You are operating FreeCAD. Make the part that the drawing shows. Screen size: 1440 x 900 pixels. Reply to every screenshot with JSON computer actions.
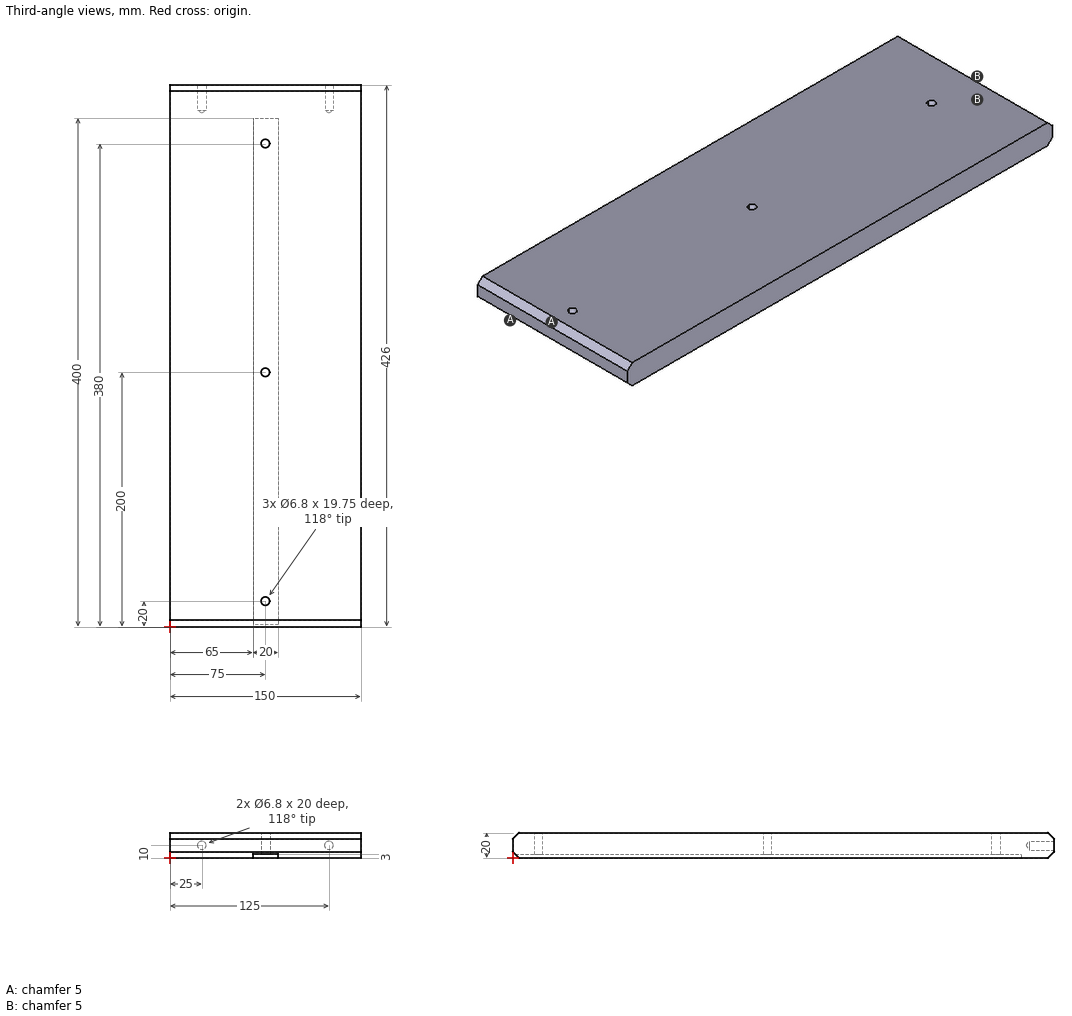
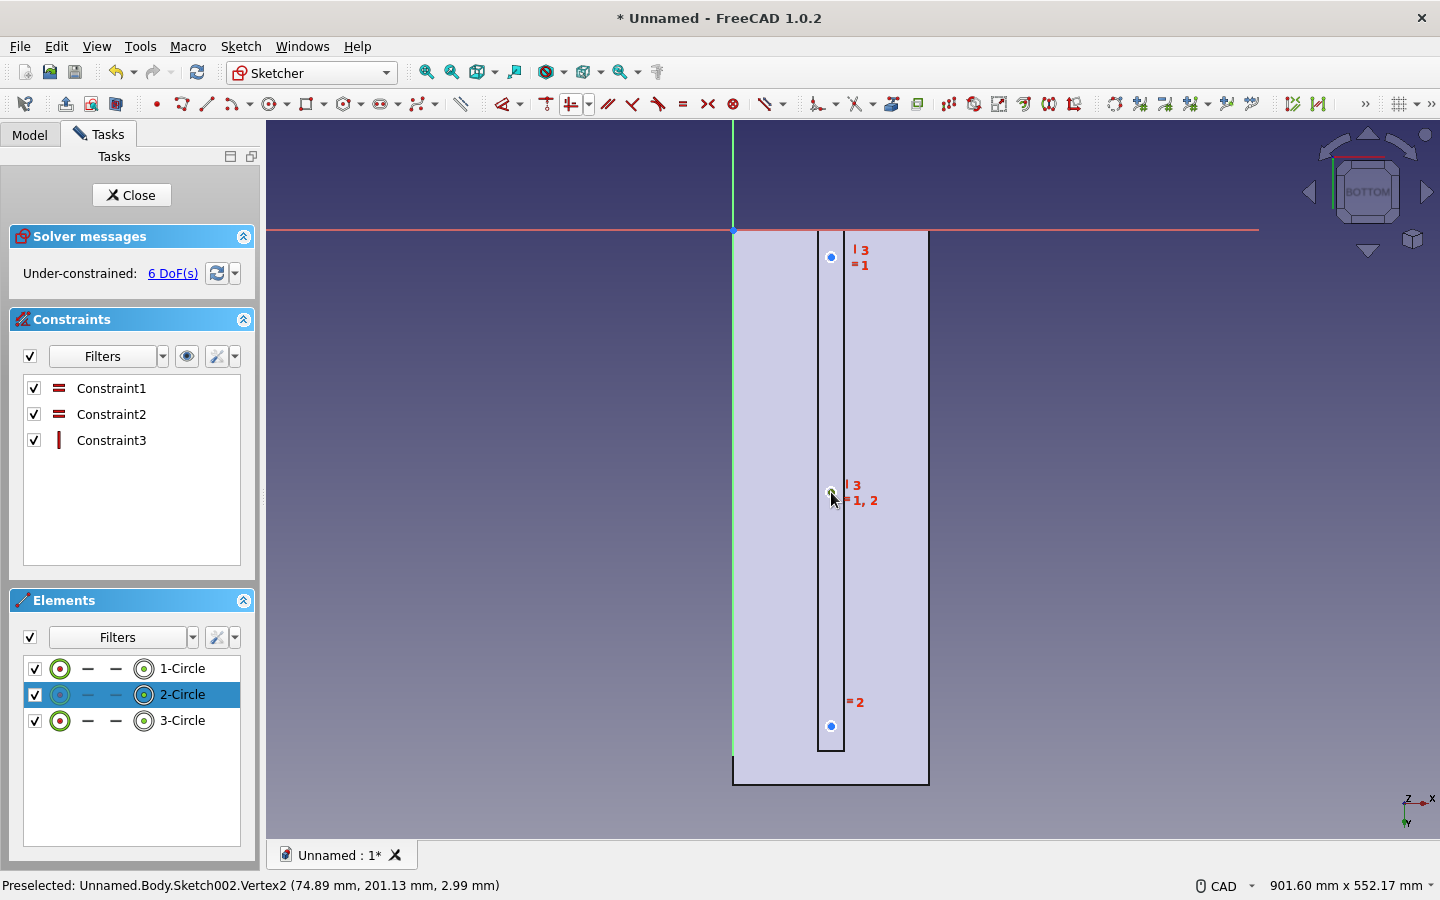
{"action": "left_click", "coordinate": [831, 726]}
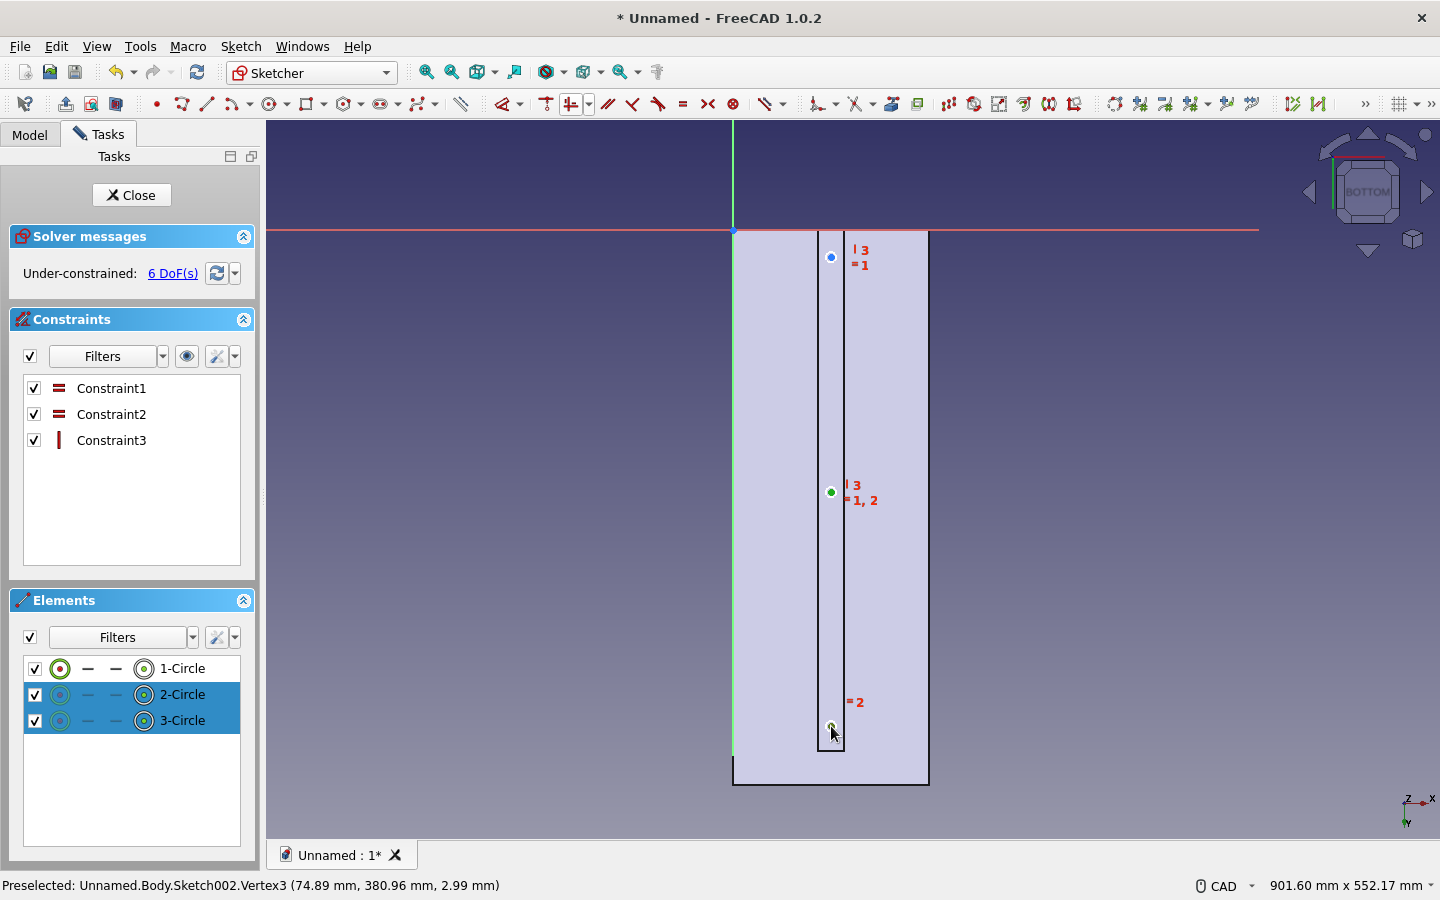
{"action": "key", "text": "v"}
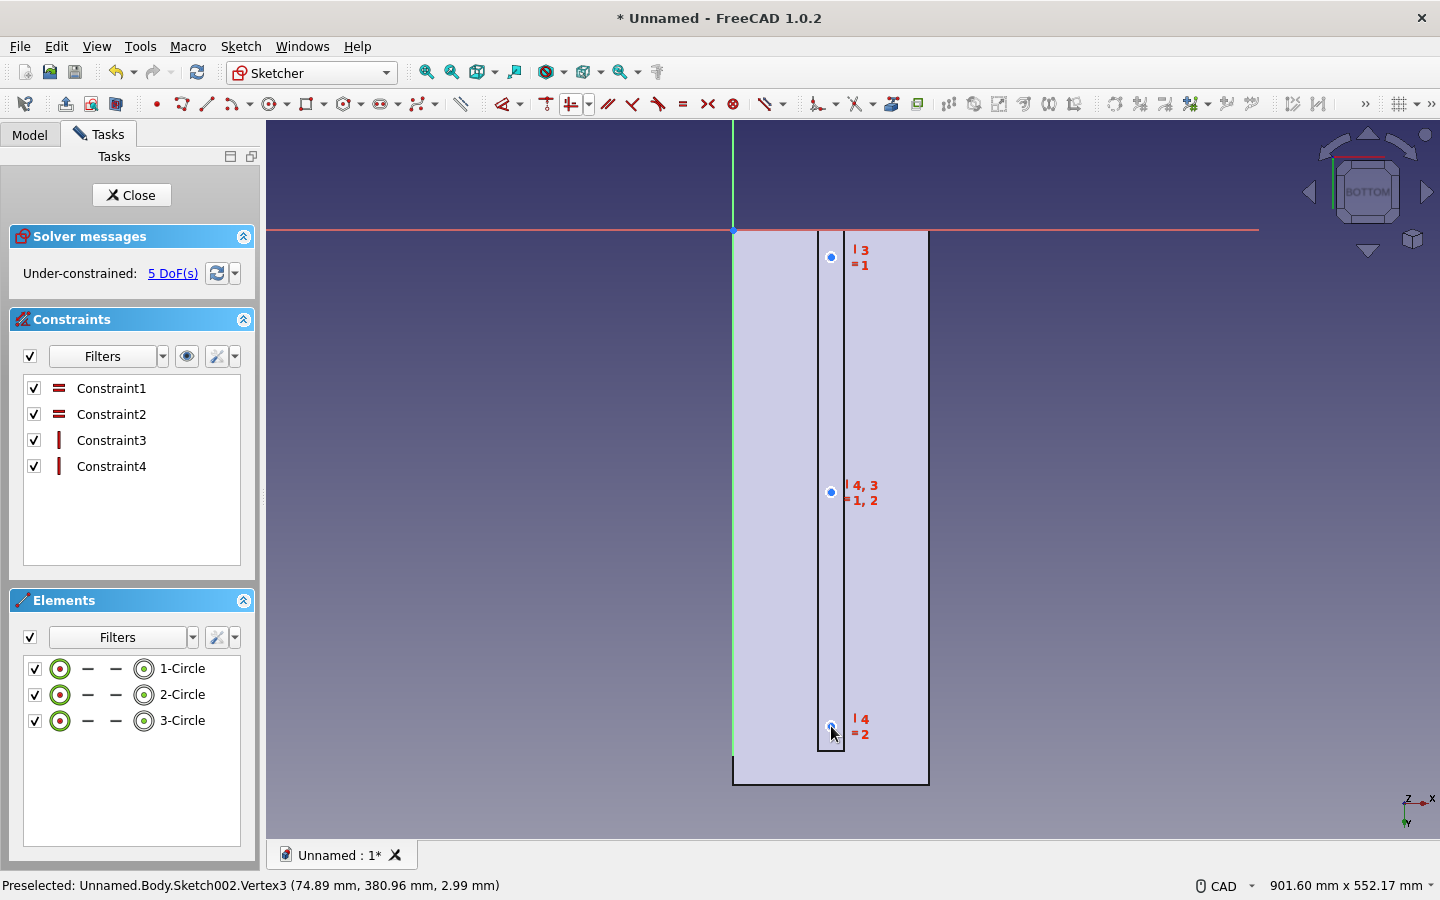
{"action": "left_click", "coordinate": [502, 104]}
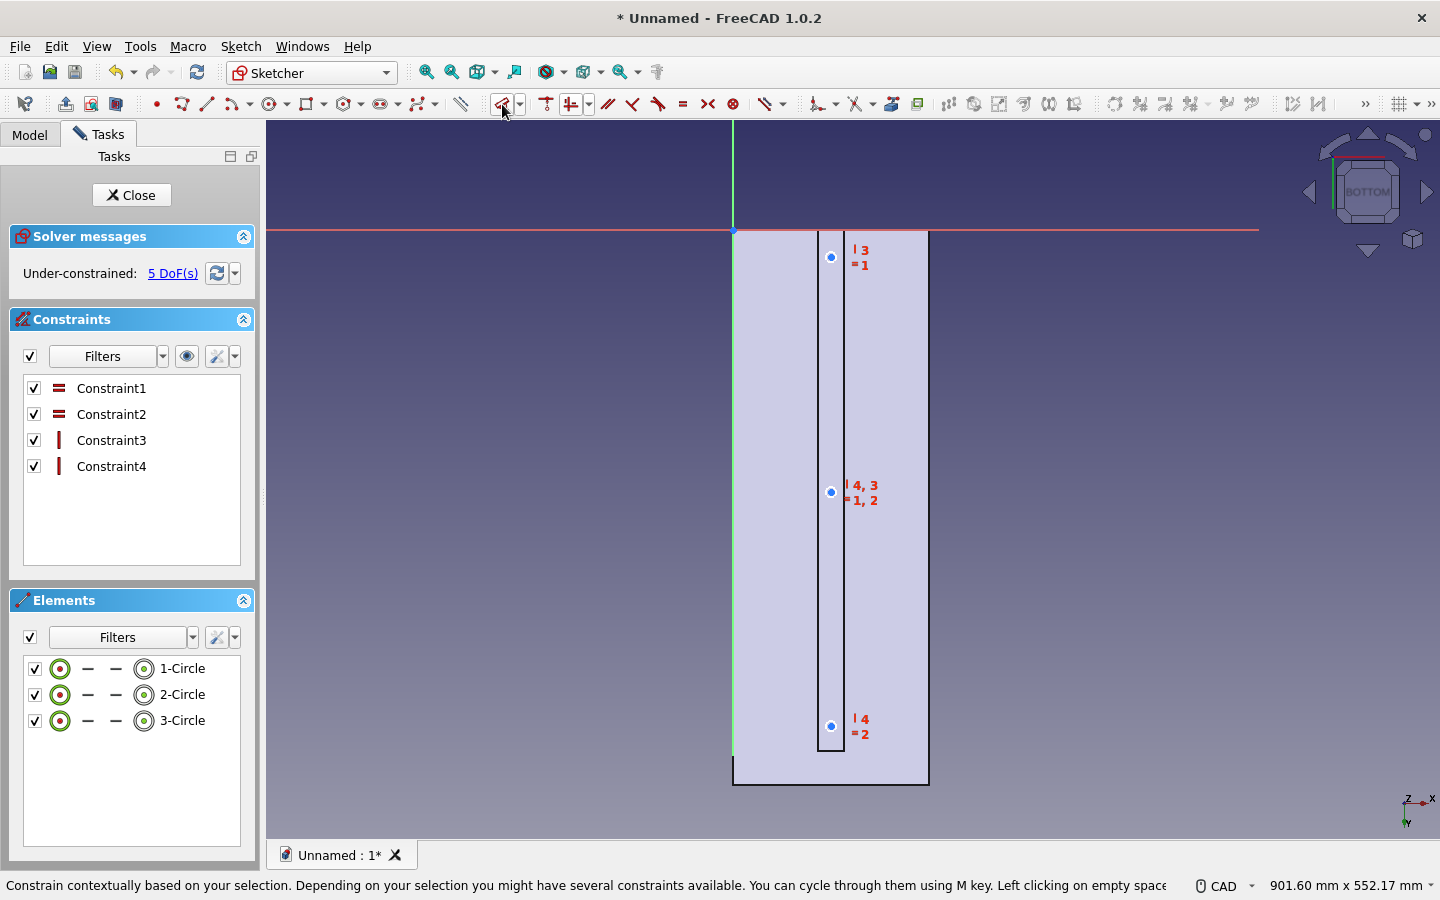
{"action": "scroll", "coordinate": [835, 261], "scroll_direction": "up", "scroll_amount": 8}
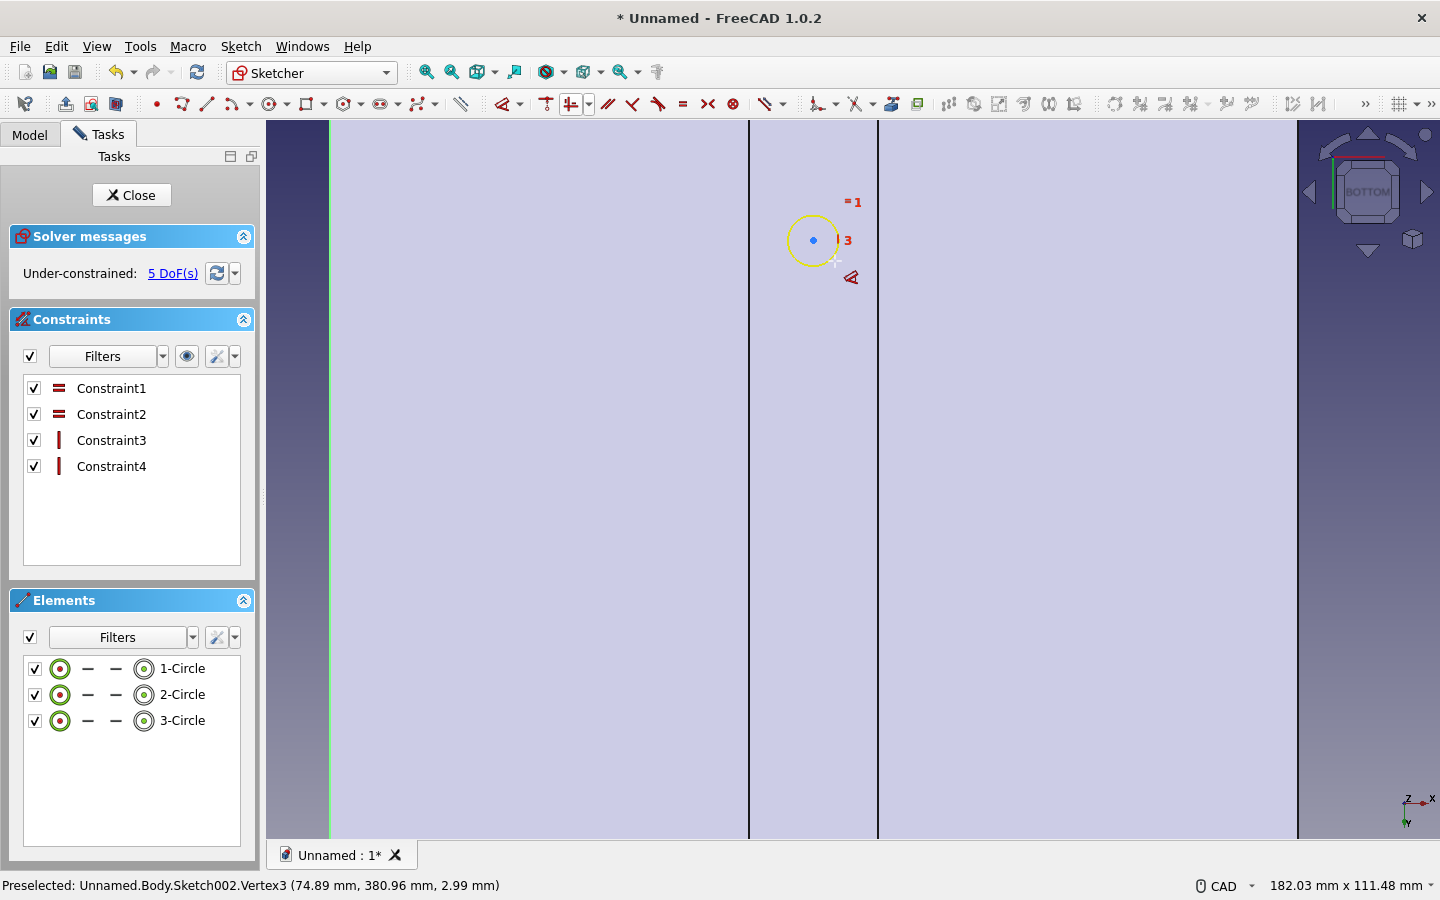
{"action": "left_click", "coordinate": [831, 259]}
{"action": "left_click", "coordinate": [853, 282]}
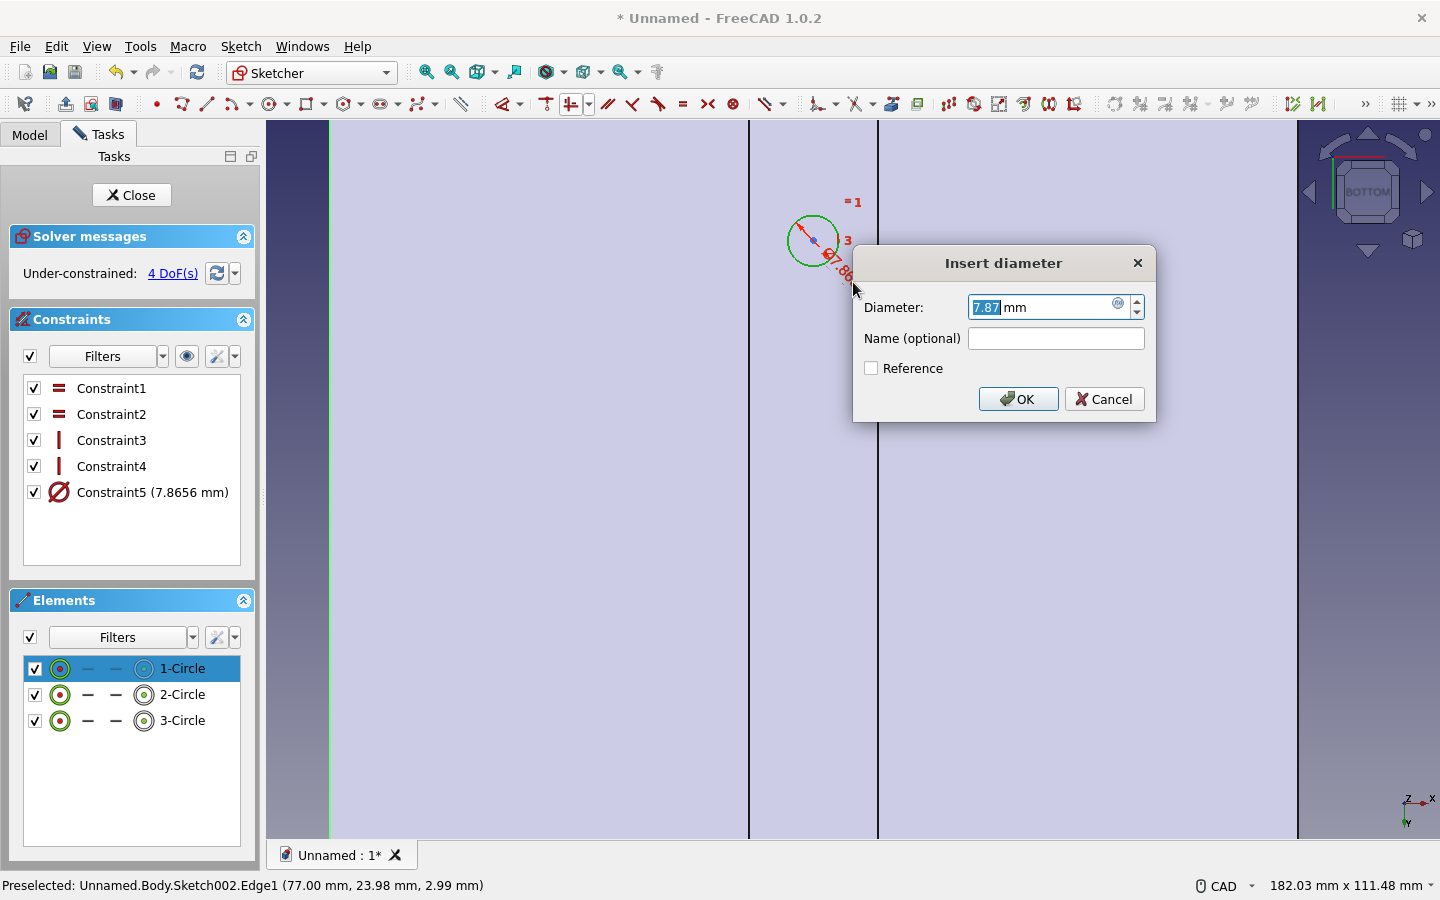
{"action": "type", "text": "6.8"}
{"action": "key", "text": "Return"}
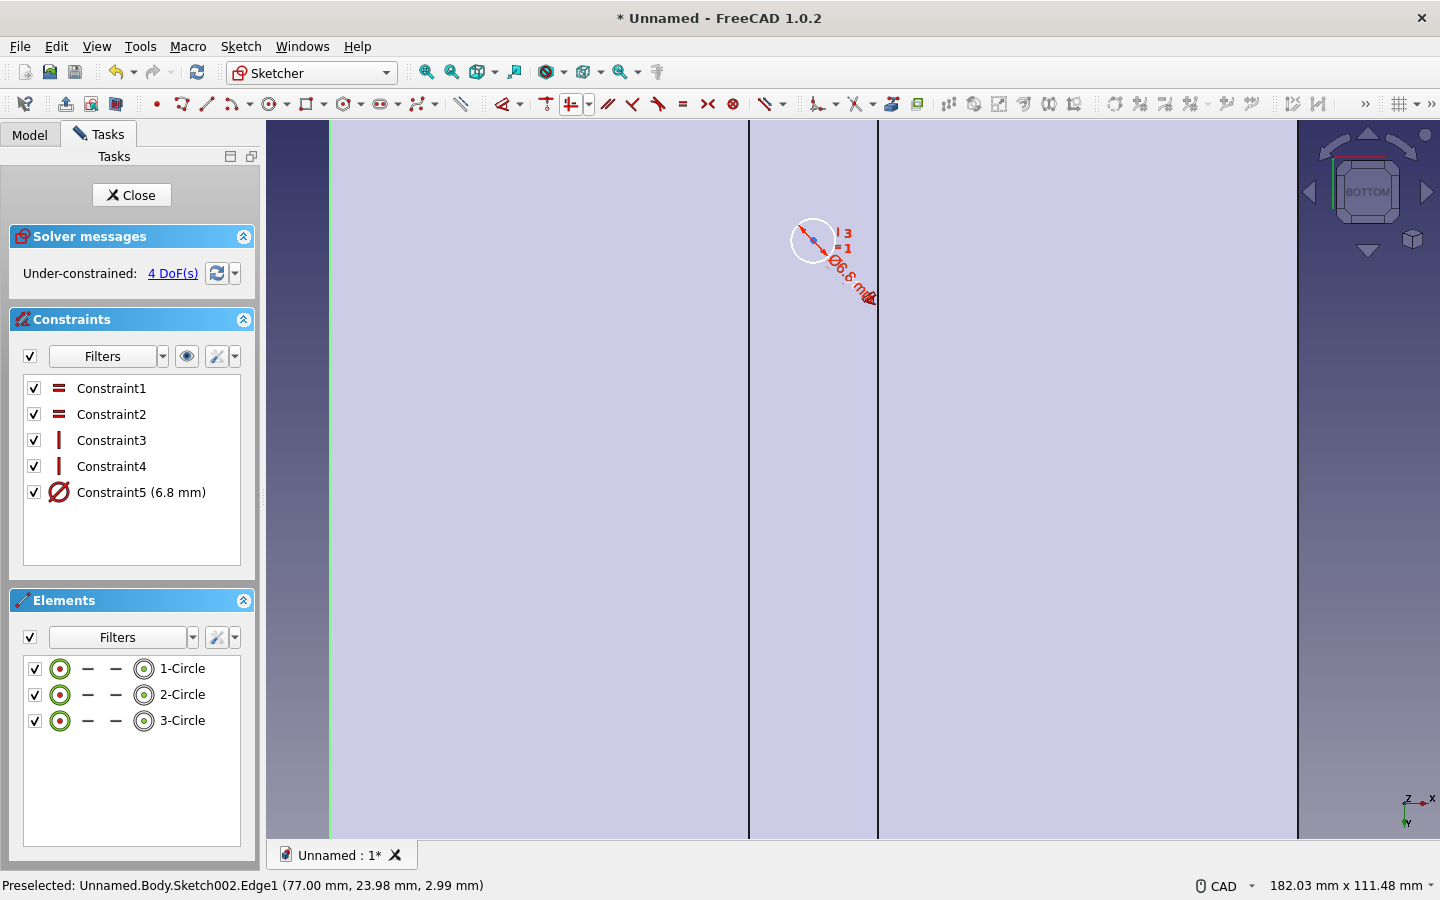
{"action": "scroll", "coordinate": [835, 261], "scroll_direction": "down", "scroll_amount": 8}